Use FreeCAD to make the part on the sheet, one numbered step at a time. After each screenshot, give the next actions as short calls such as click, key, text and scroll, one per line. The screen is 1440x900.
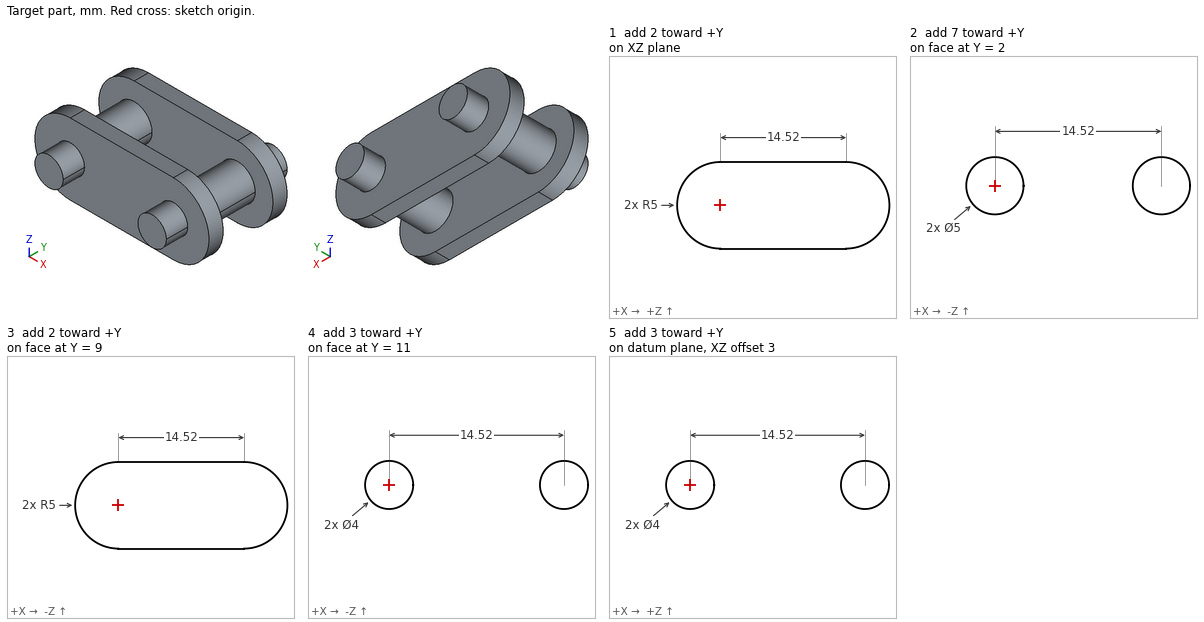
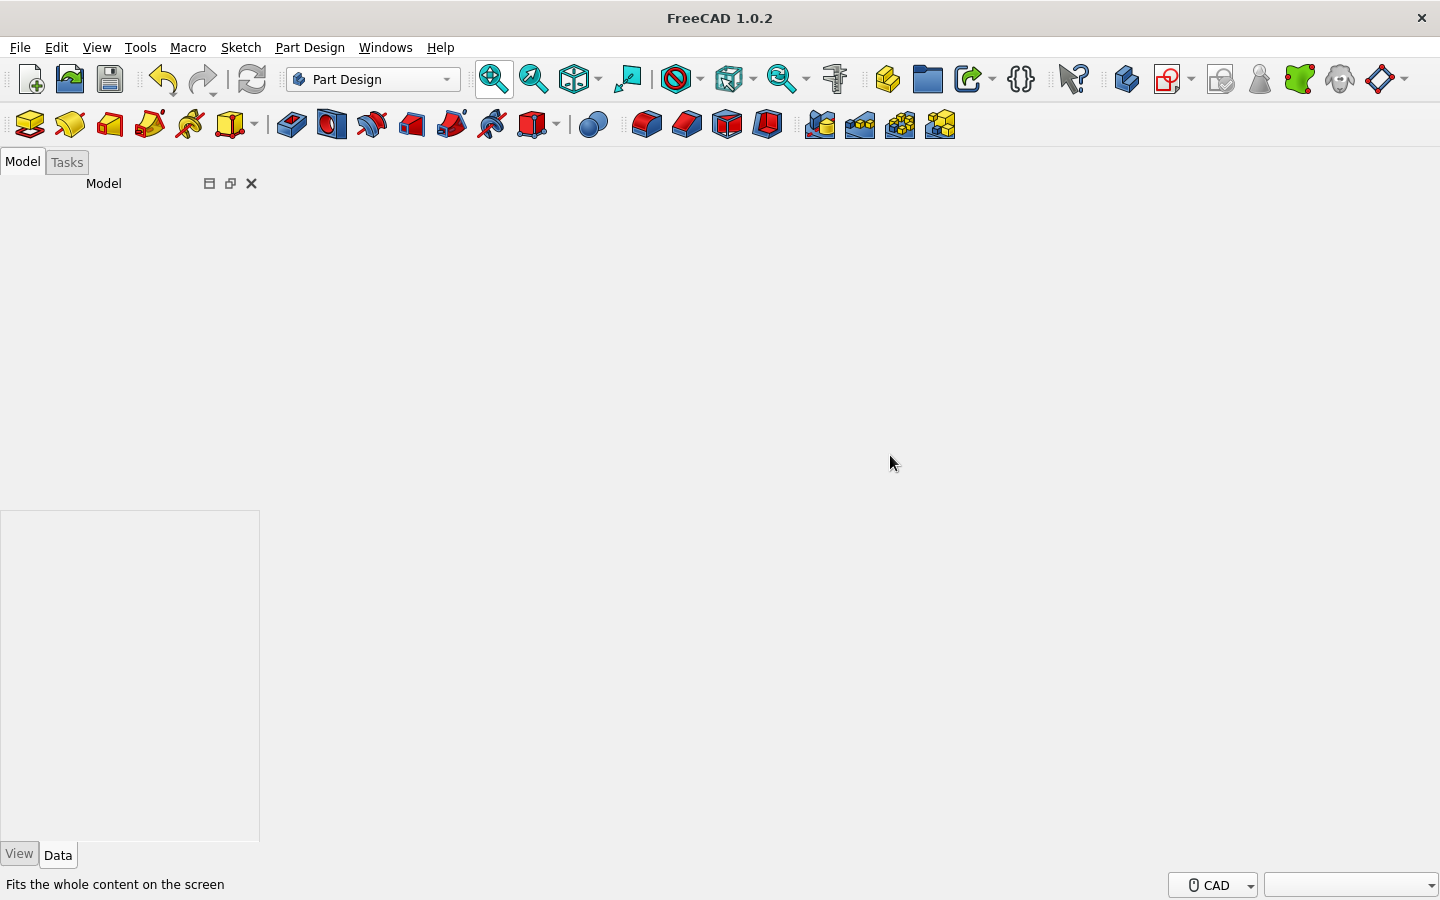
key(ctrl+n)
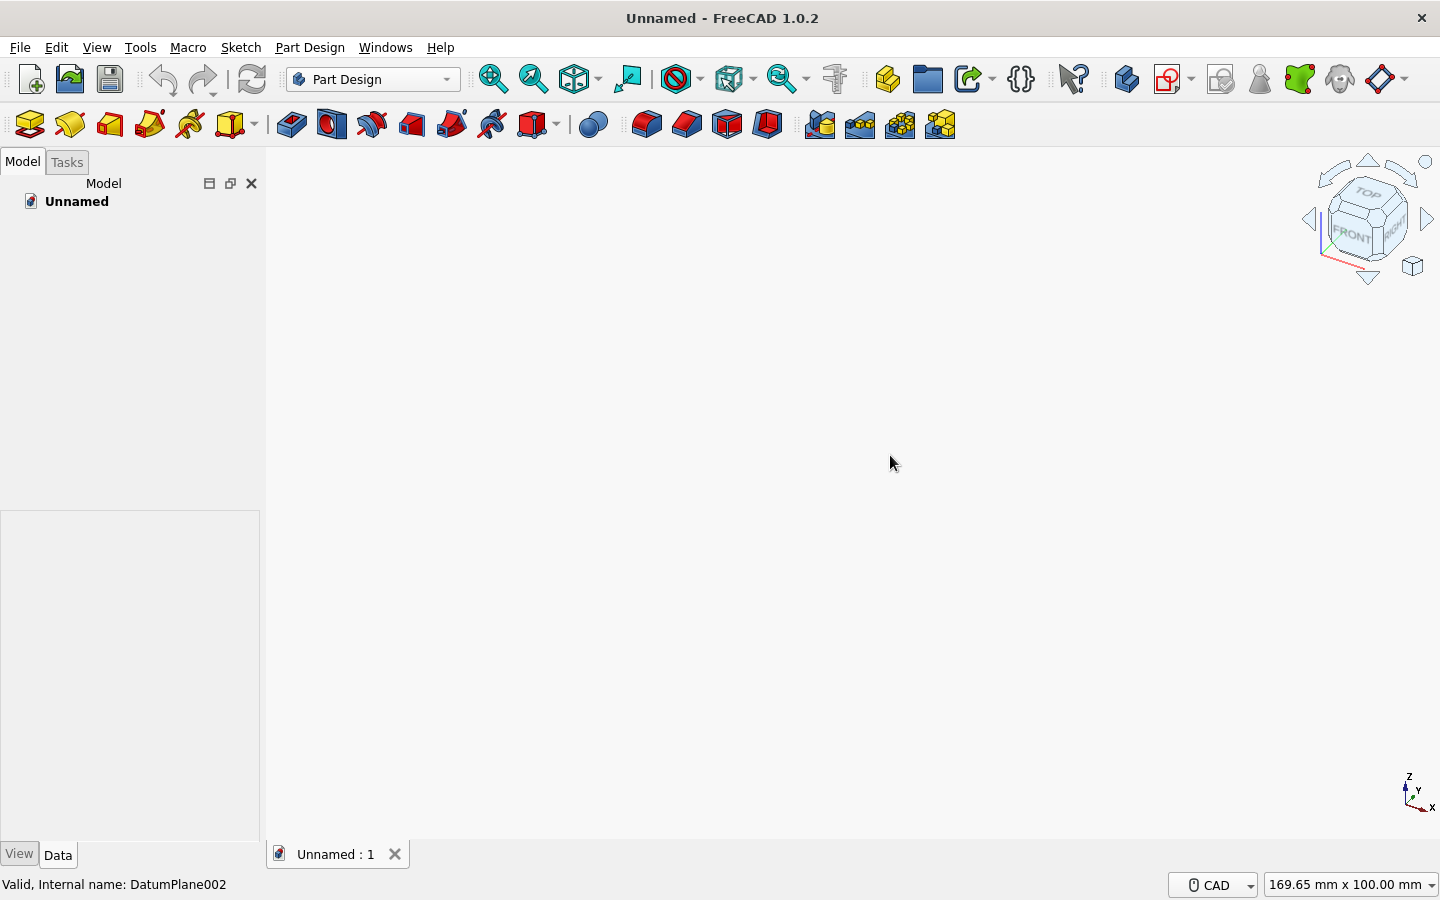
click(1168, 80)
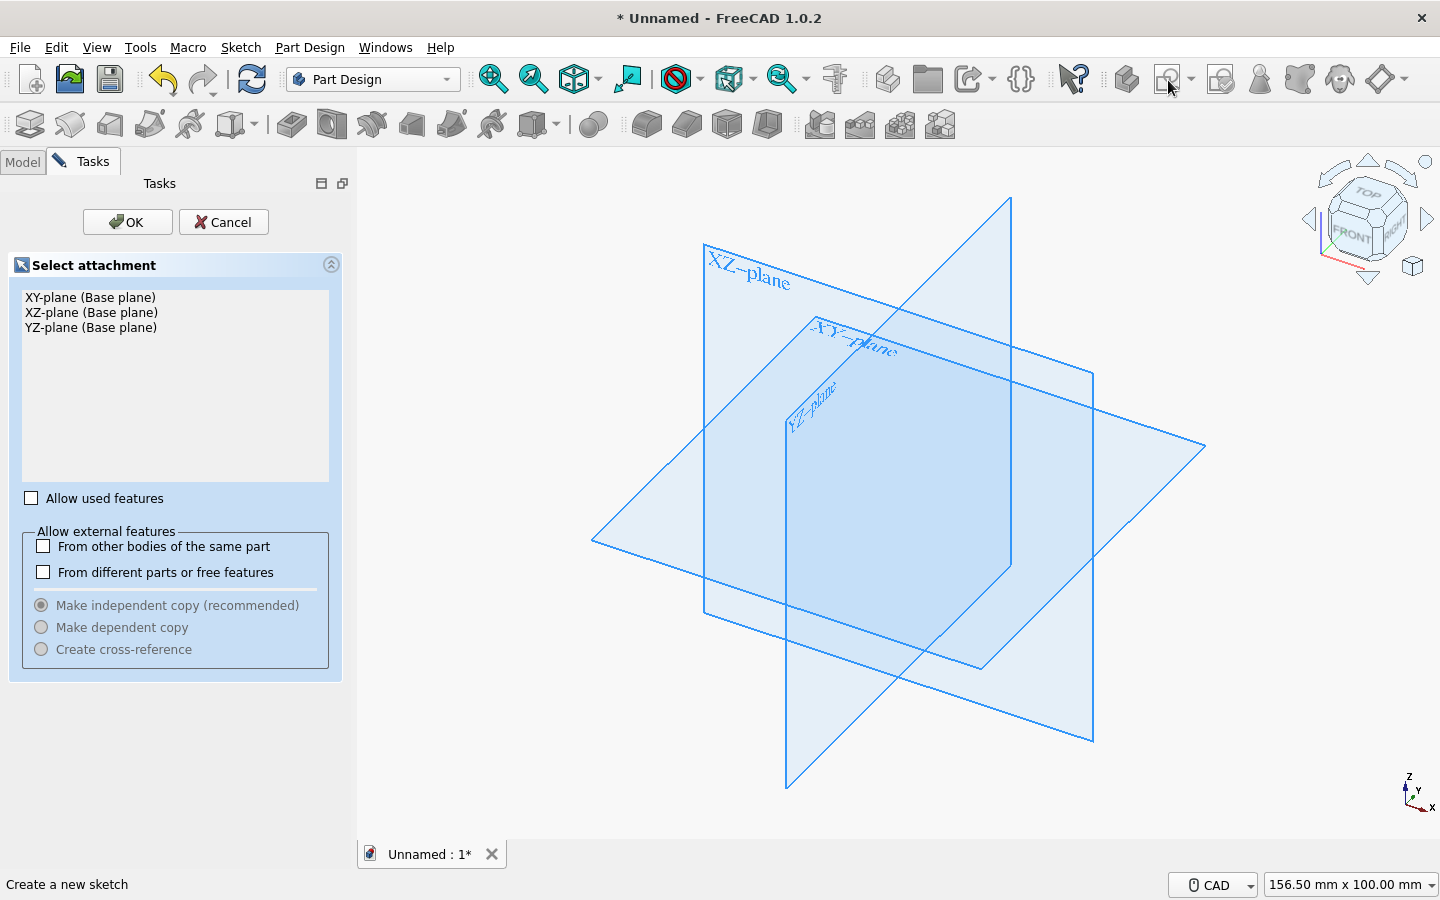
click(82, 312)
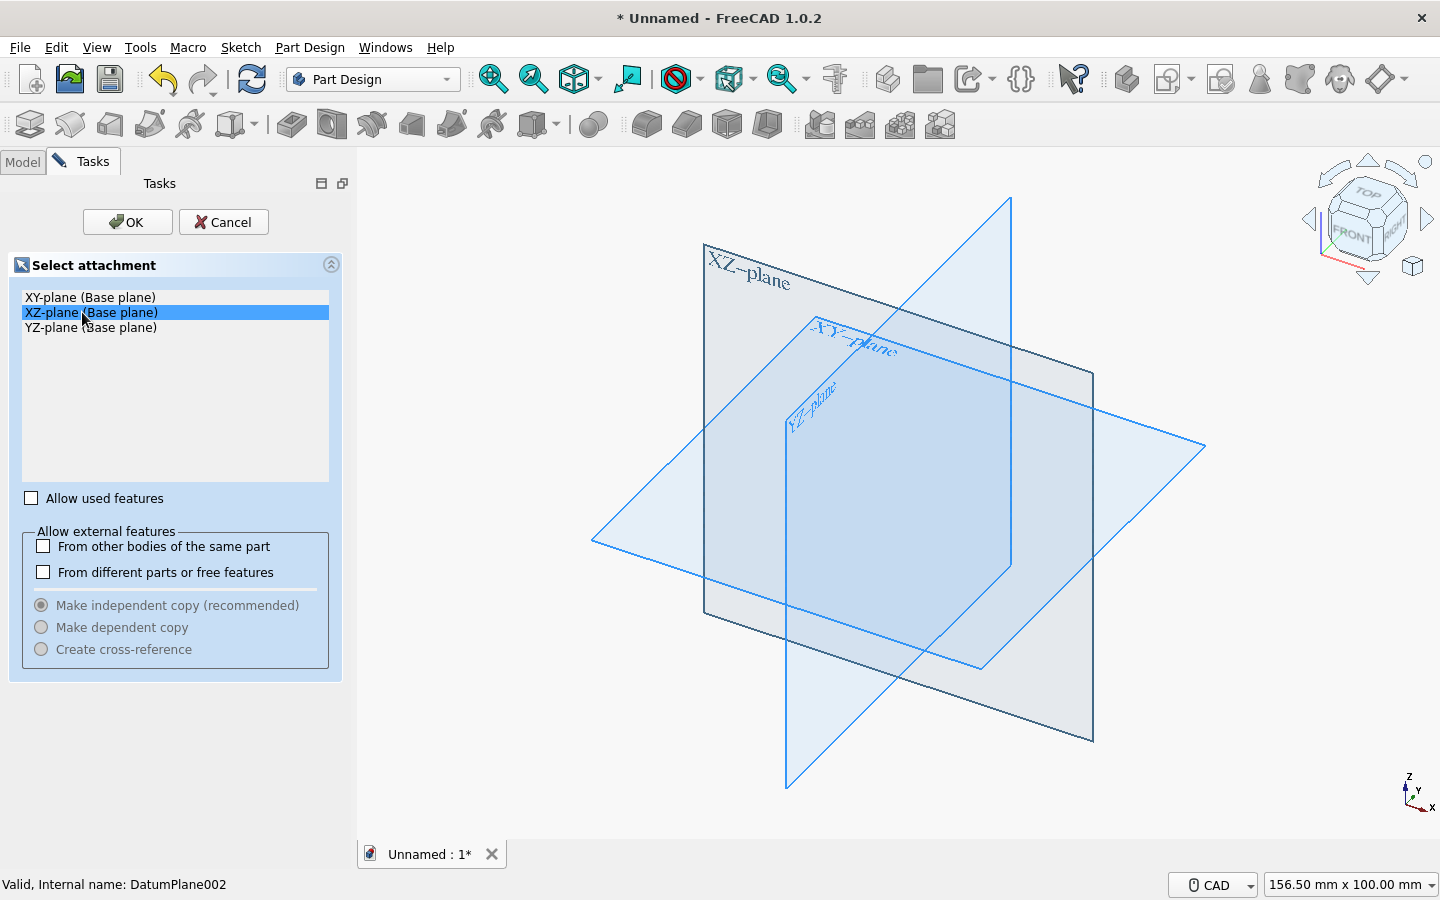
click(128, 222)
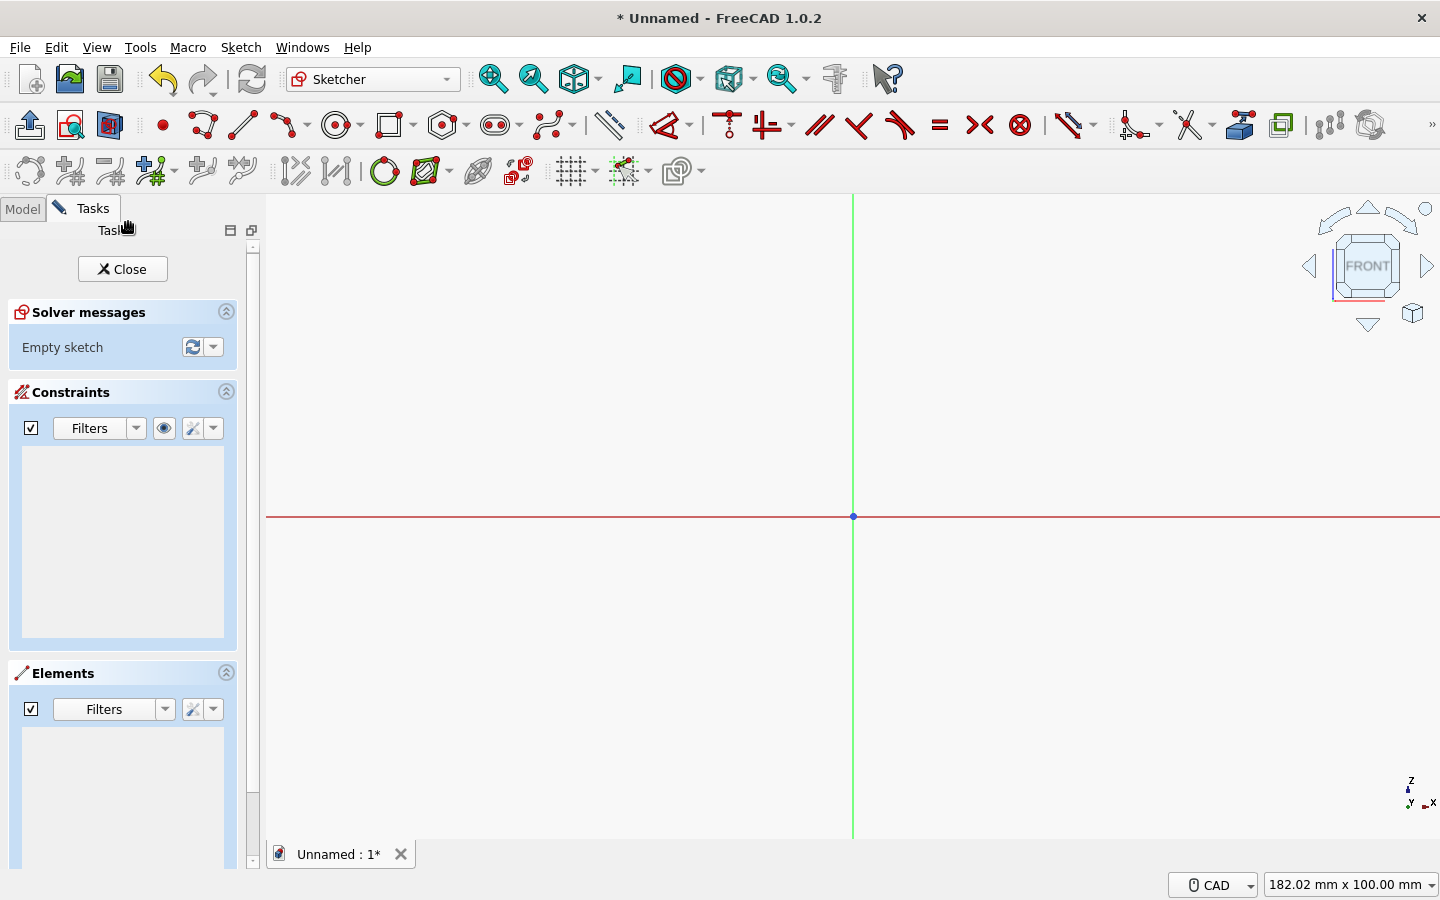
scroll(938, 516, up, 7)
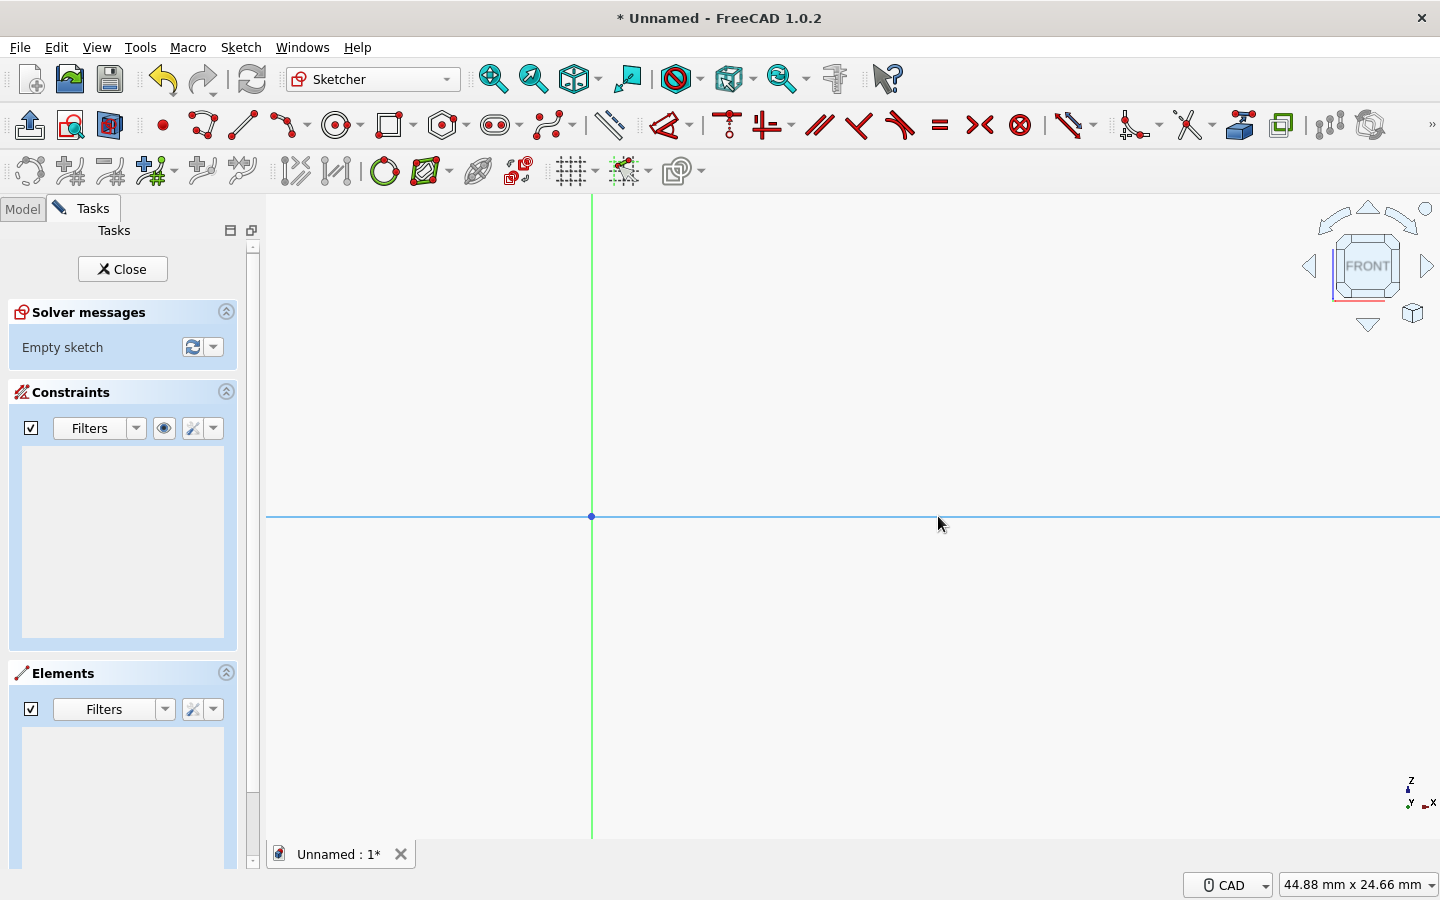
key(g)
key(s)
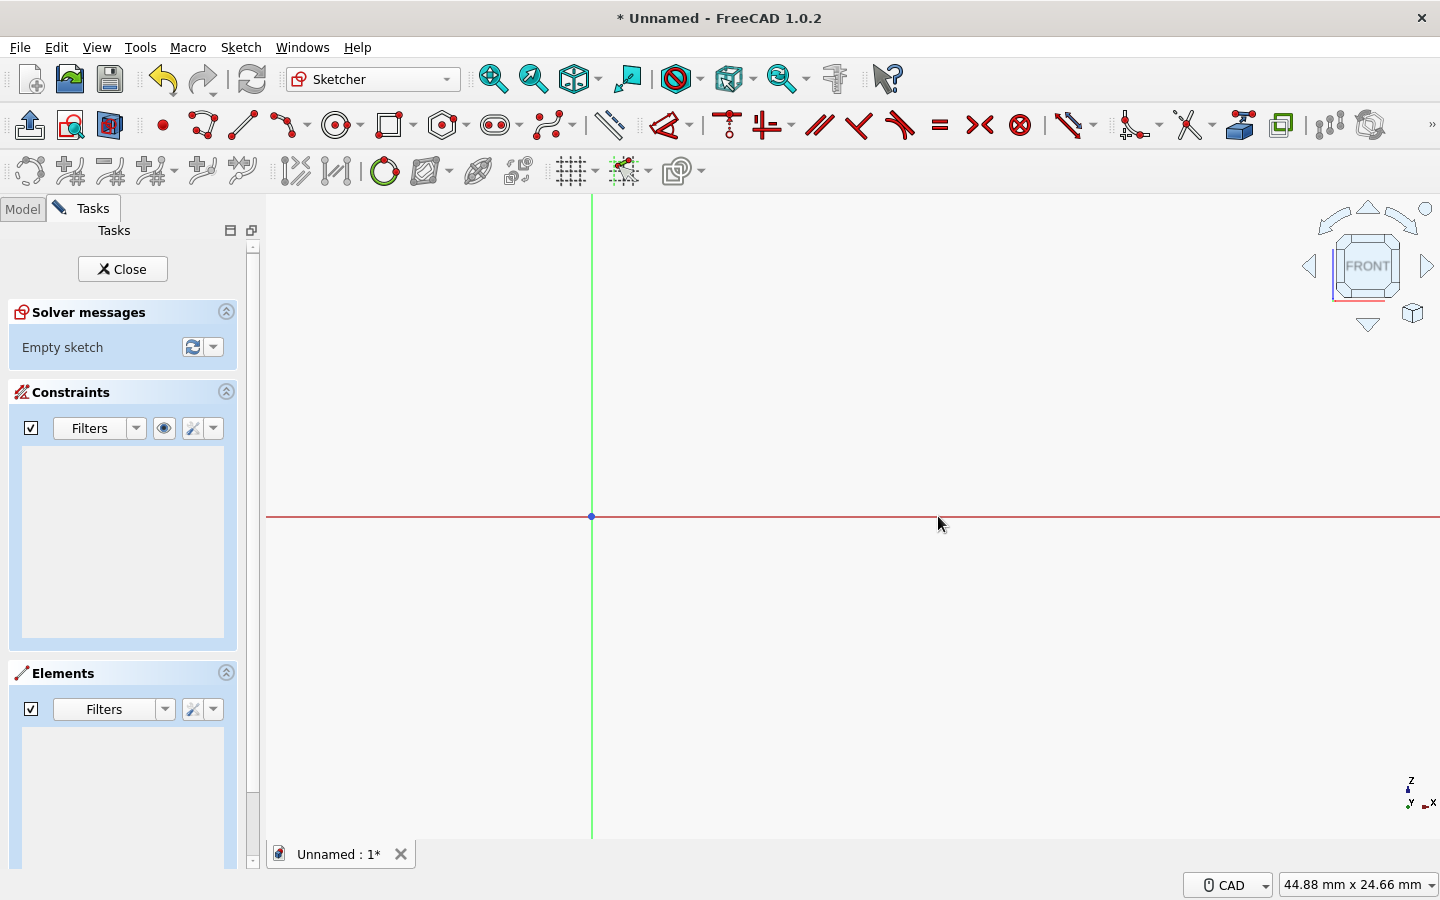
click(592, 516)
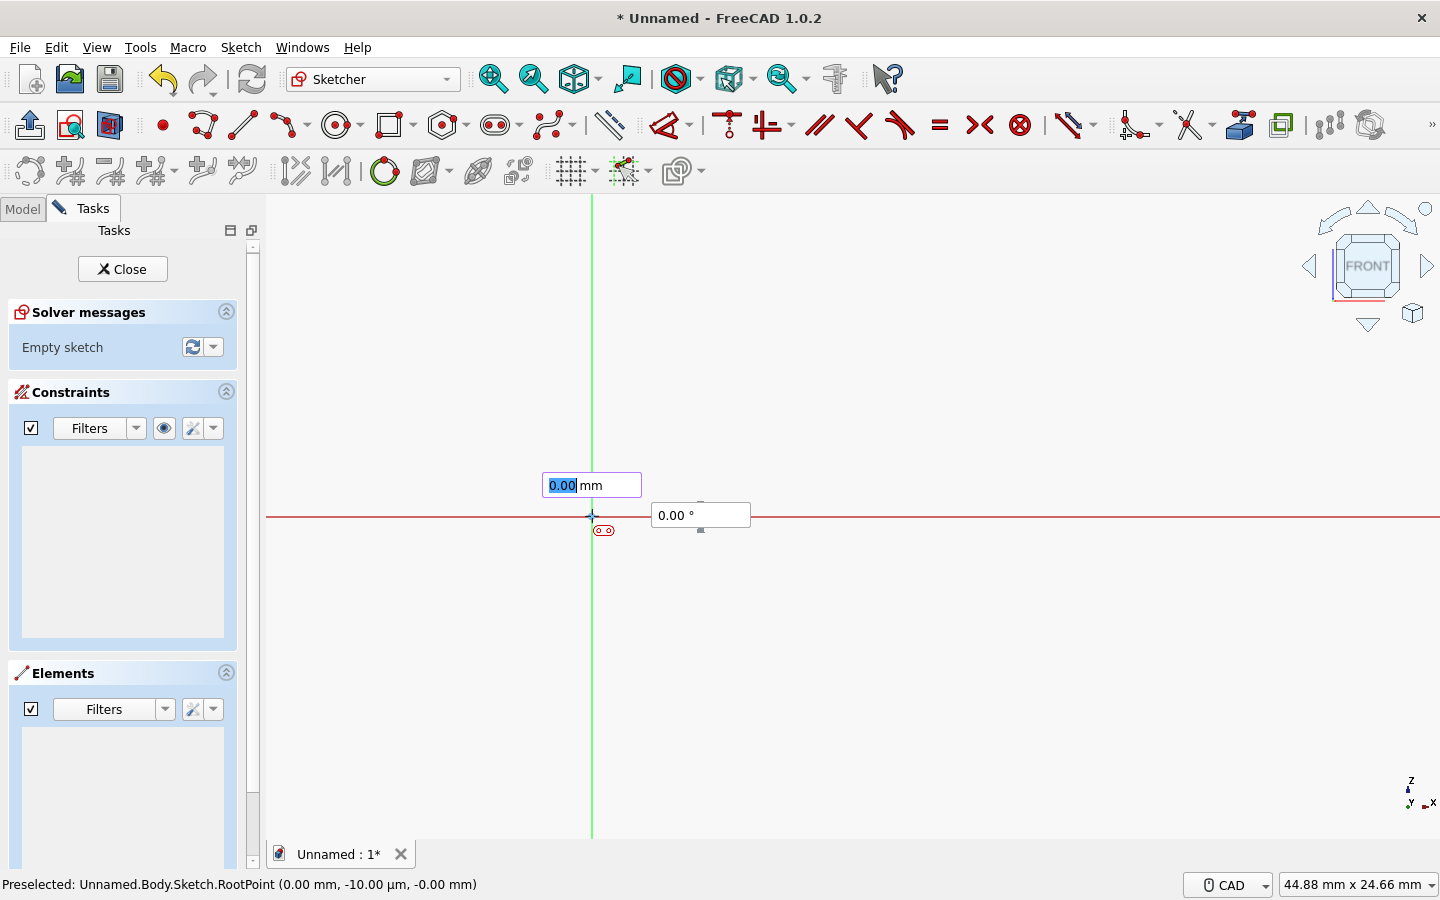
click(971, 508)